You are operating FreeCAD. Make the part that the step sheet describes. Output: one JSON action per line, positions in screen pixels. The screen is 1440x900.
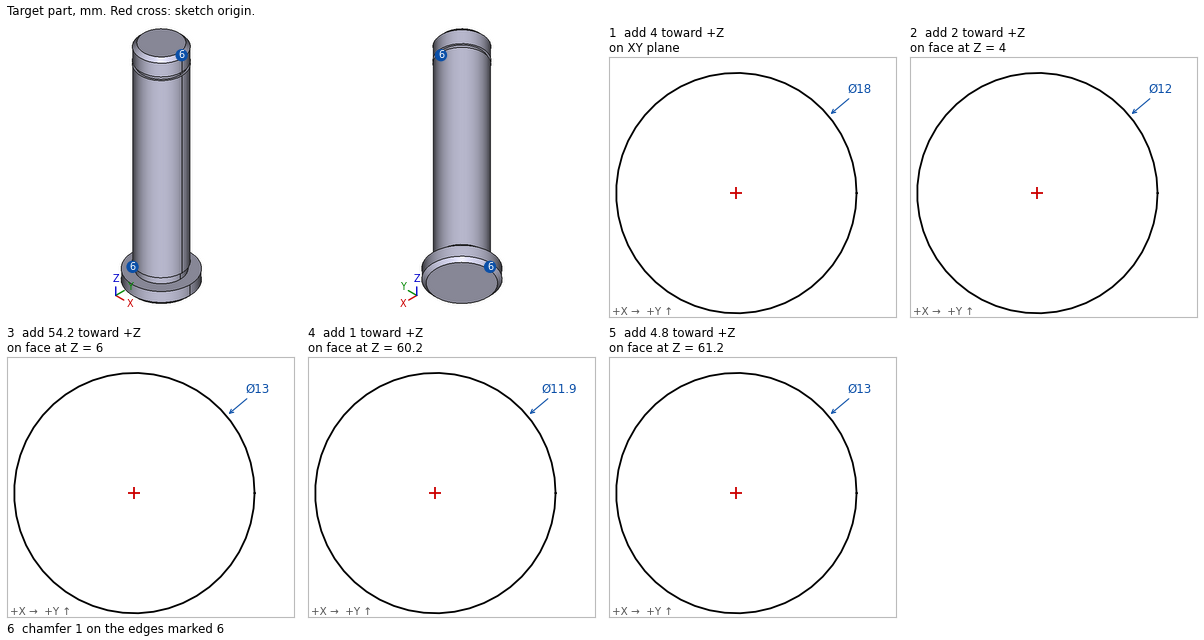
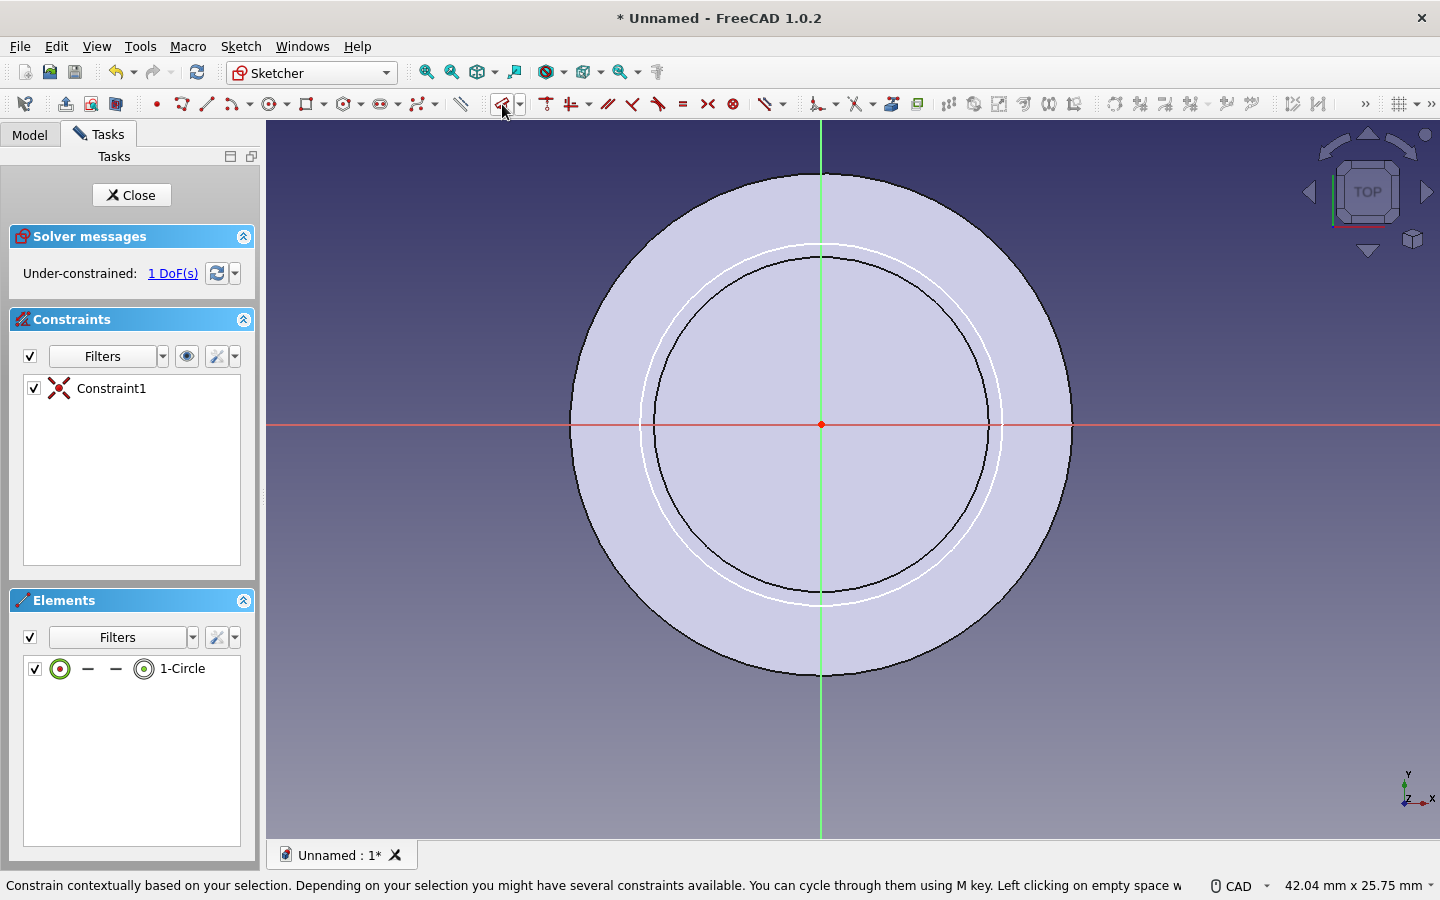
{"action": "left_click", "coordinate": [949, 296]}
{"action": "left_click", "coordinate": [972, 273]}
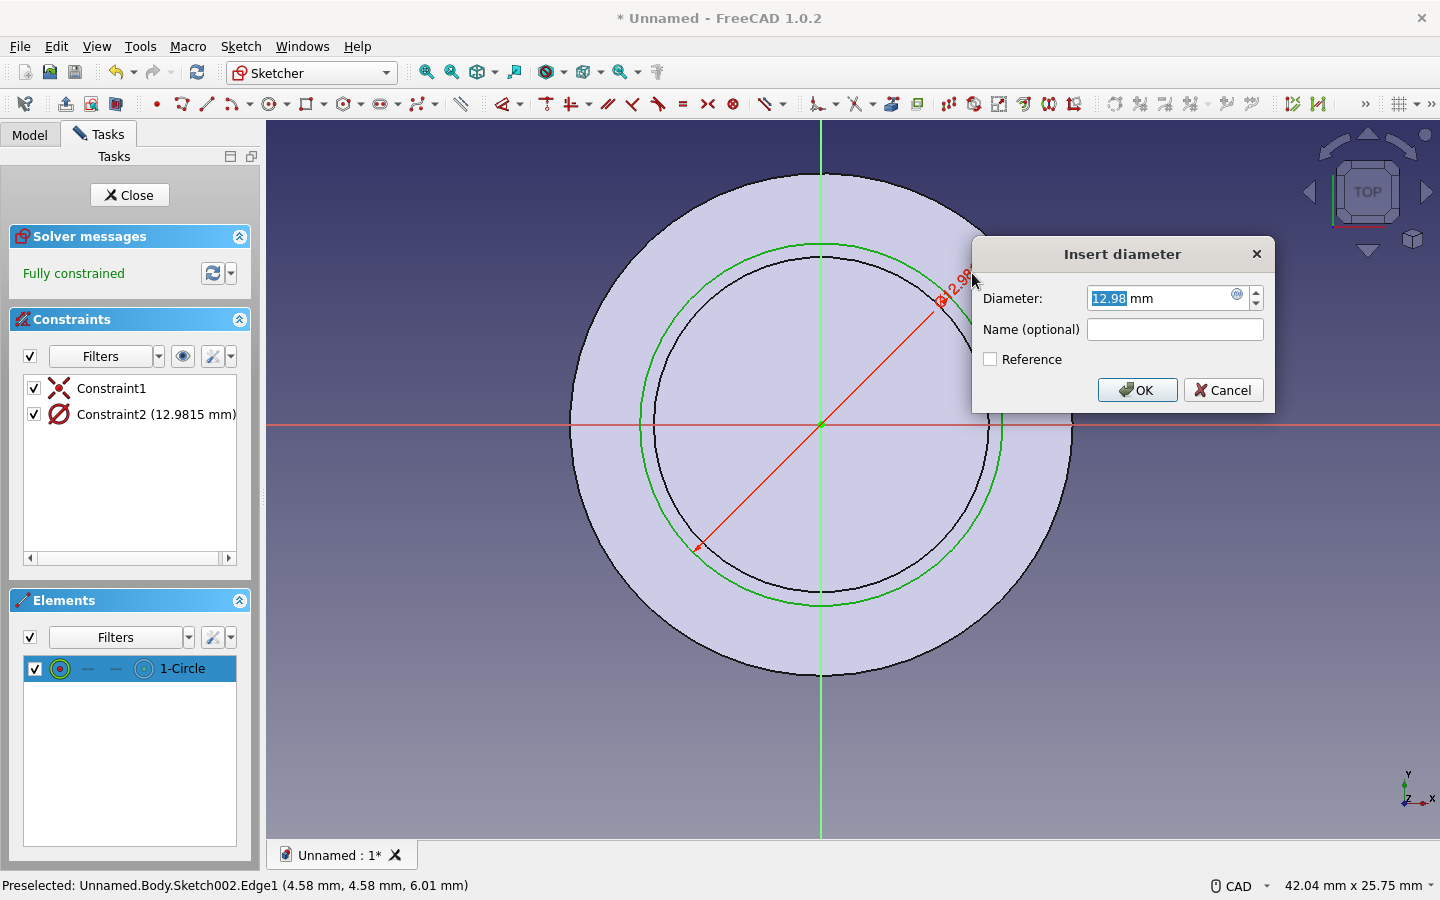
{"action": "type", "text": "13"}
{"action": "key", "text": "Return"}
{"action": "key", "text": "Escape"}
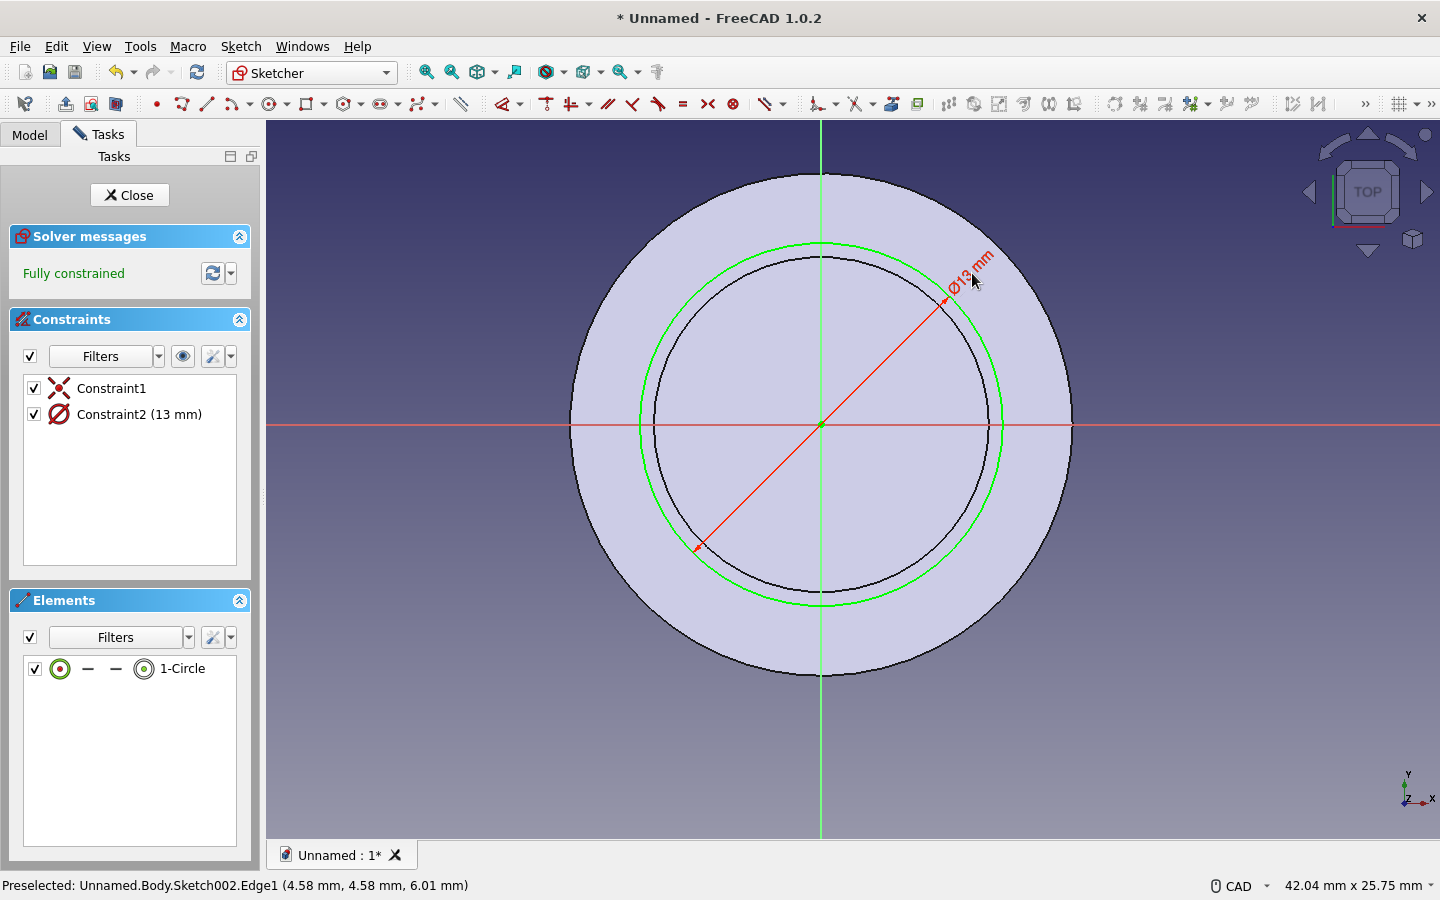
{"action": "left_click", "coordinate": [130, 195]}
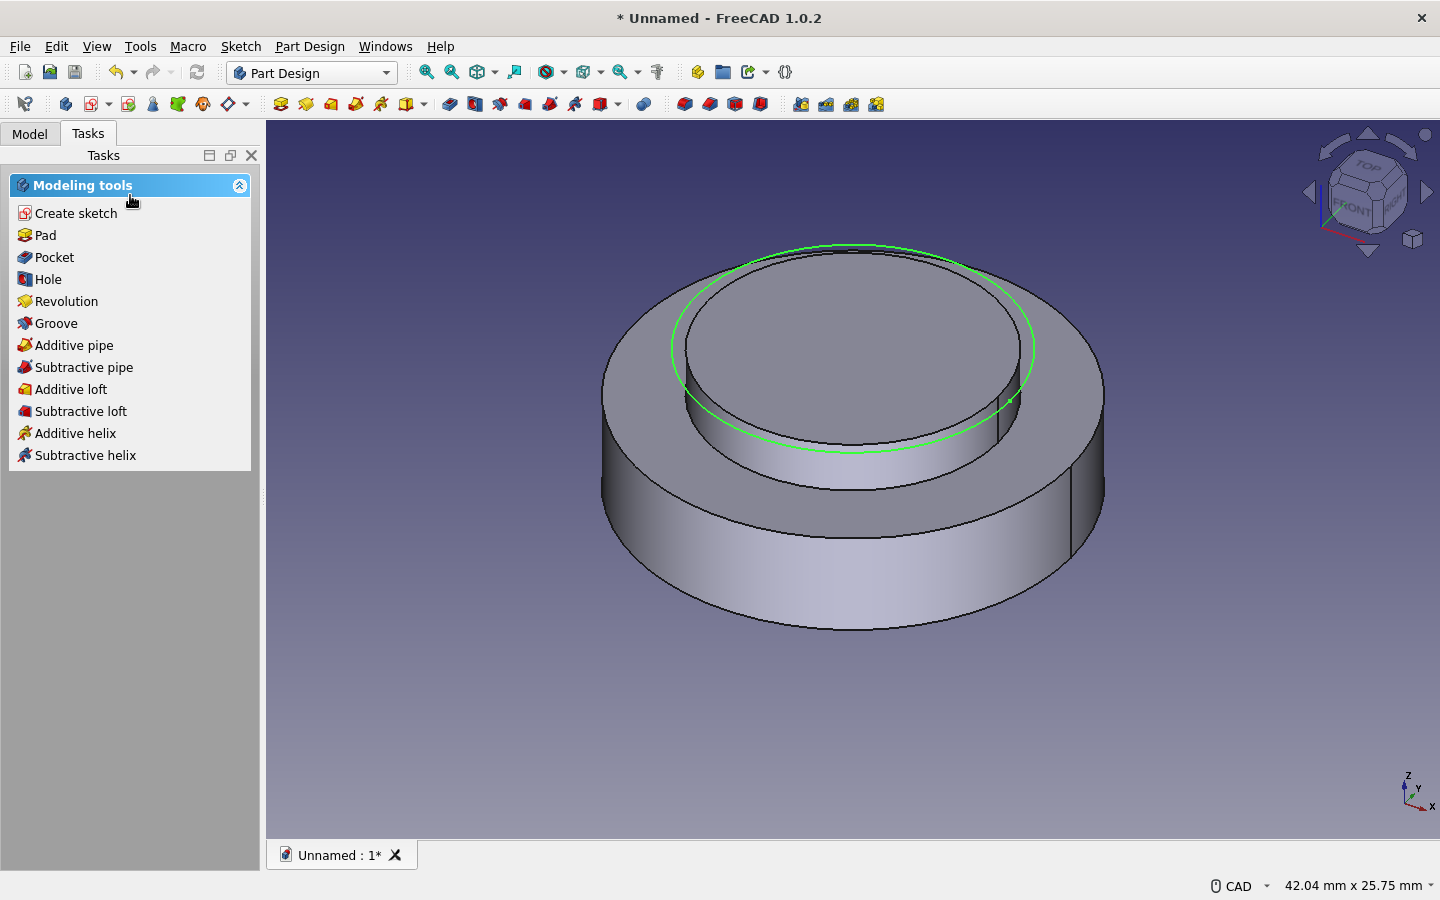
{"action": "left_click", "coordinate": [281, 104]}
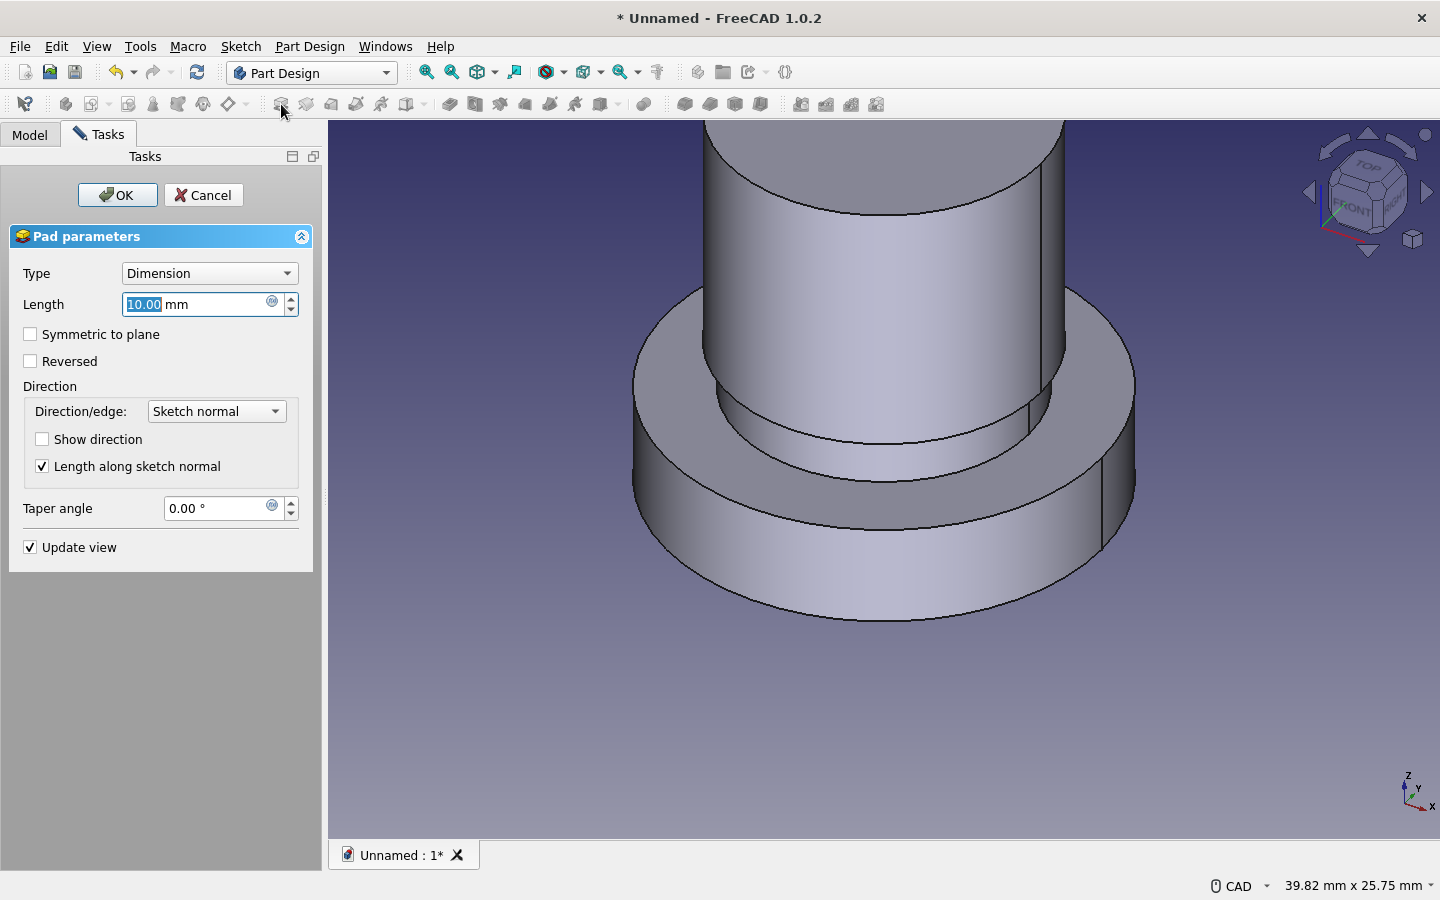
{"action": "type", "text": "54.2"}
{"action": "key", "text": "Tab"}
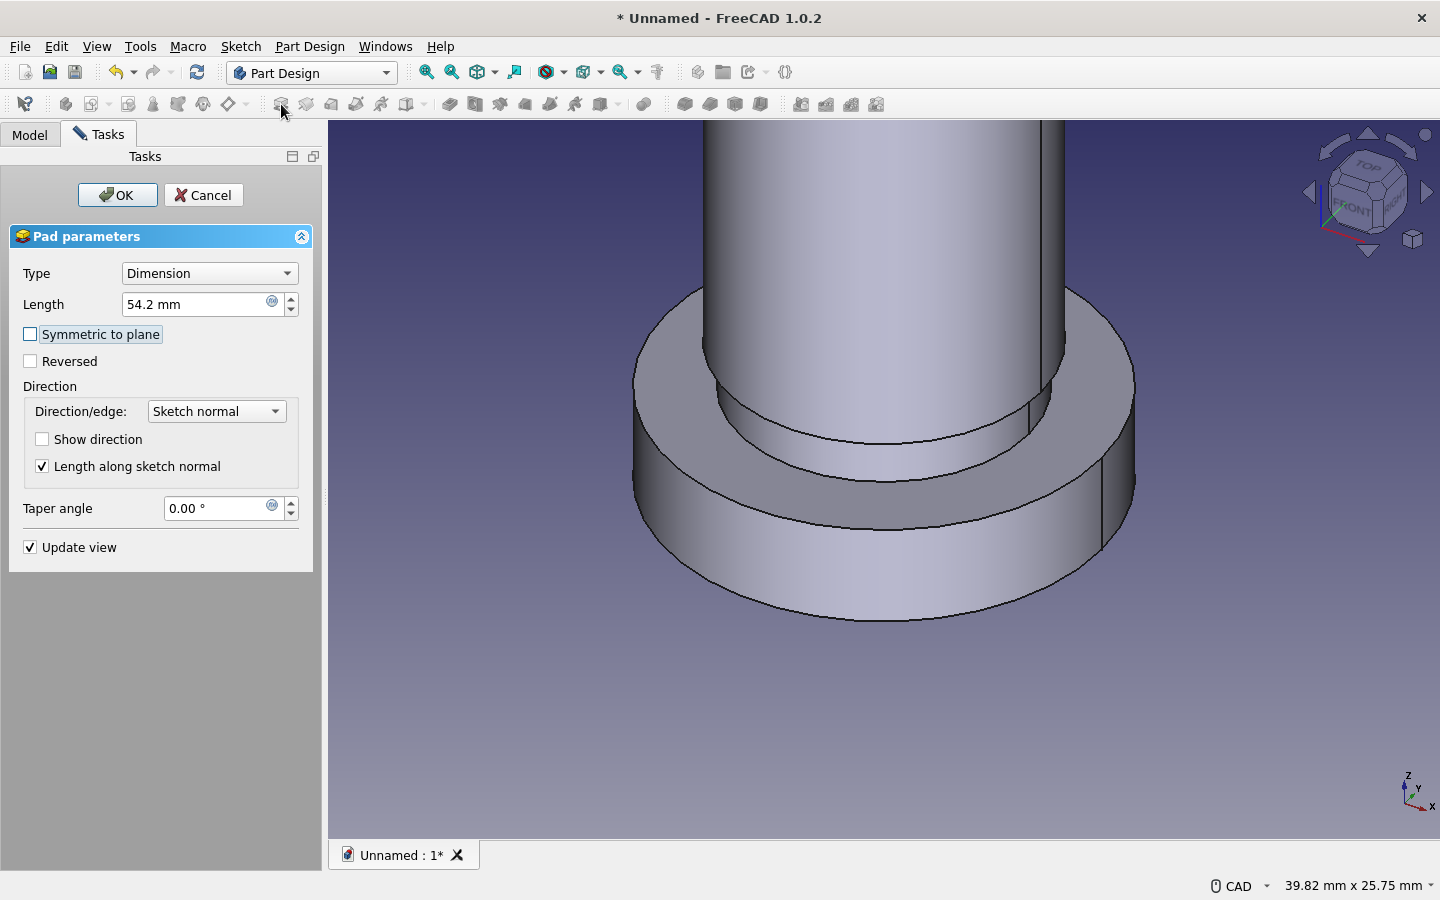
{"action": "left_click", "coordinate": [118, 195]}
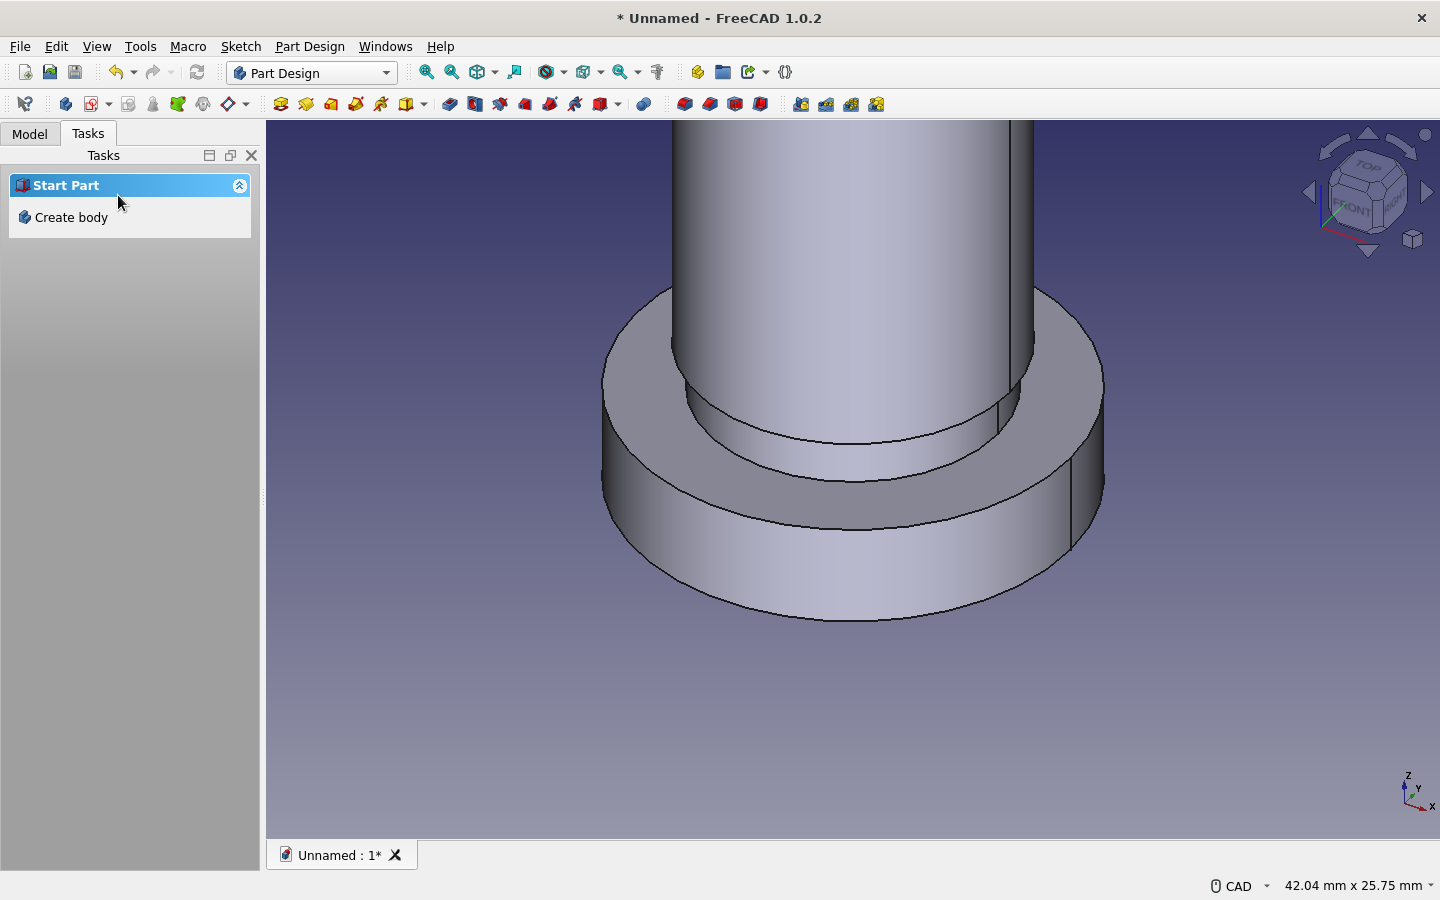
{"action": "left_click", "coordinate": [427, 72]}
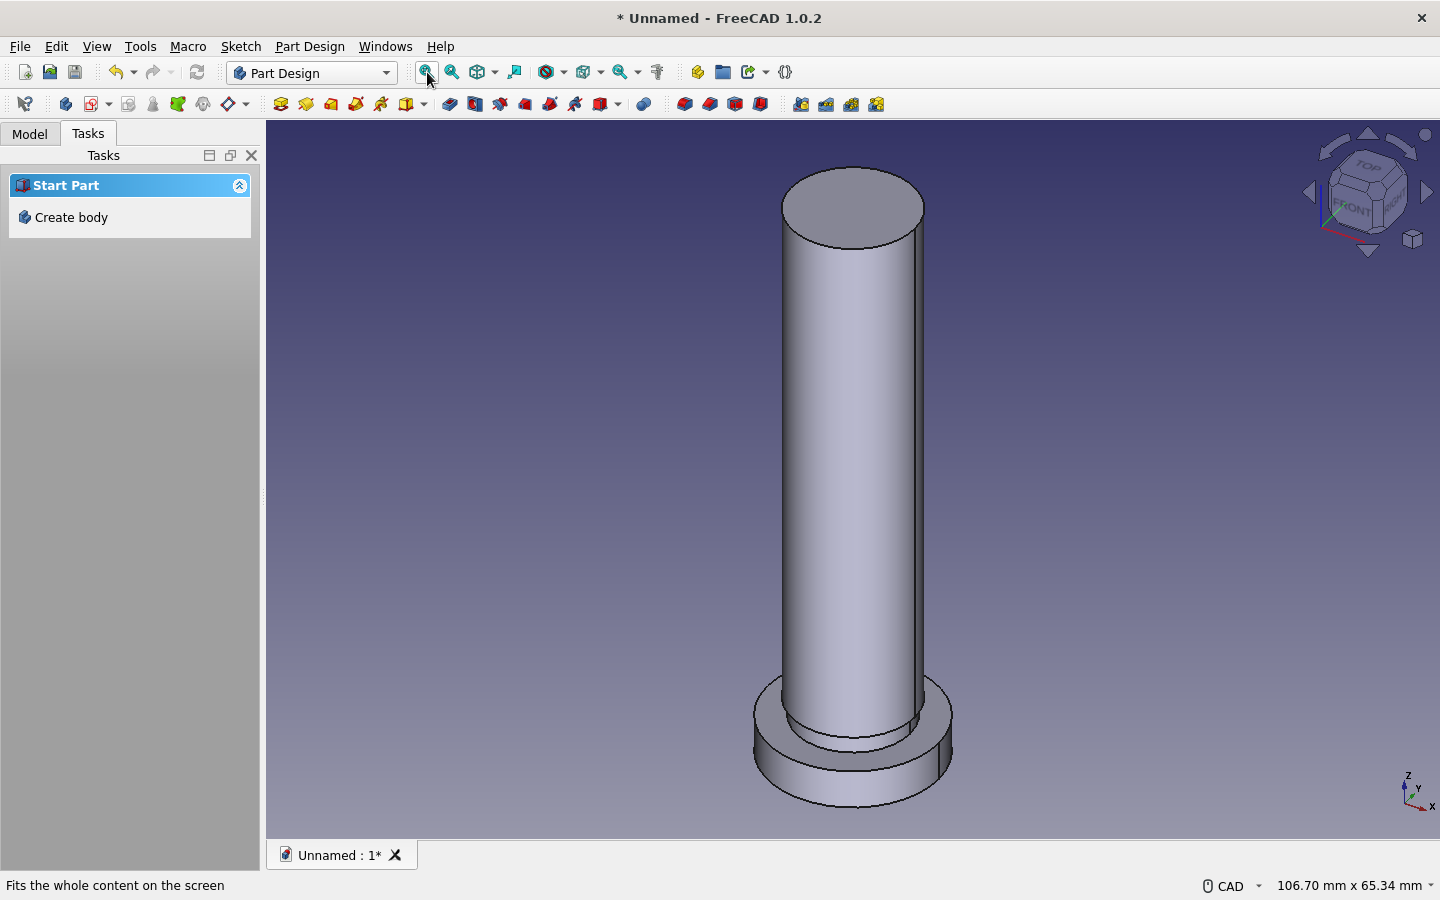
{"action": "left_click", "coordinate": [853, 207]}